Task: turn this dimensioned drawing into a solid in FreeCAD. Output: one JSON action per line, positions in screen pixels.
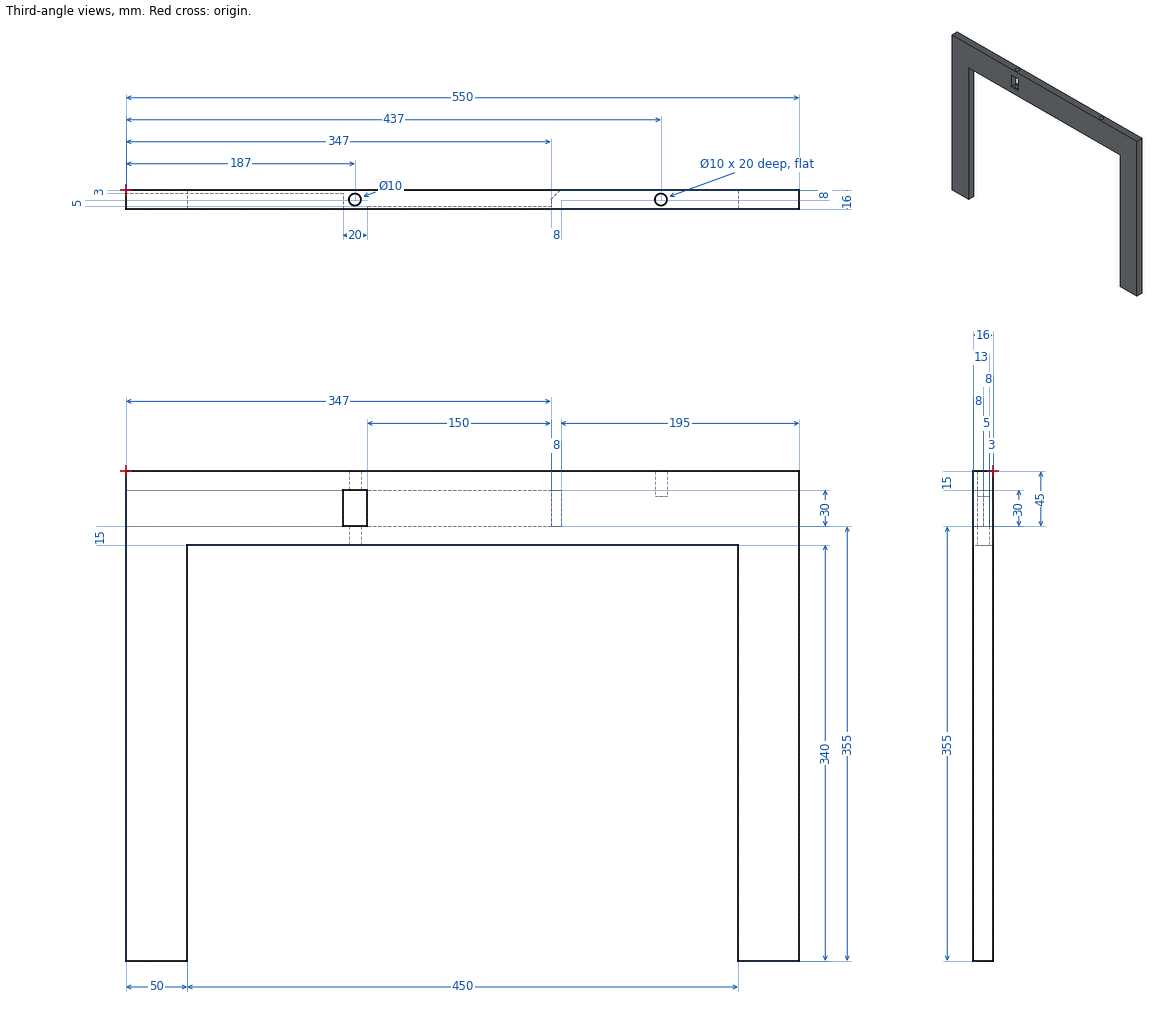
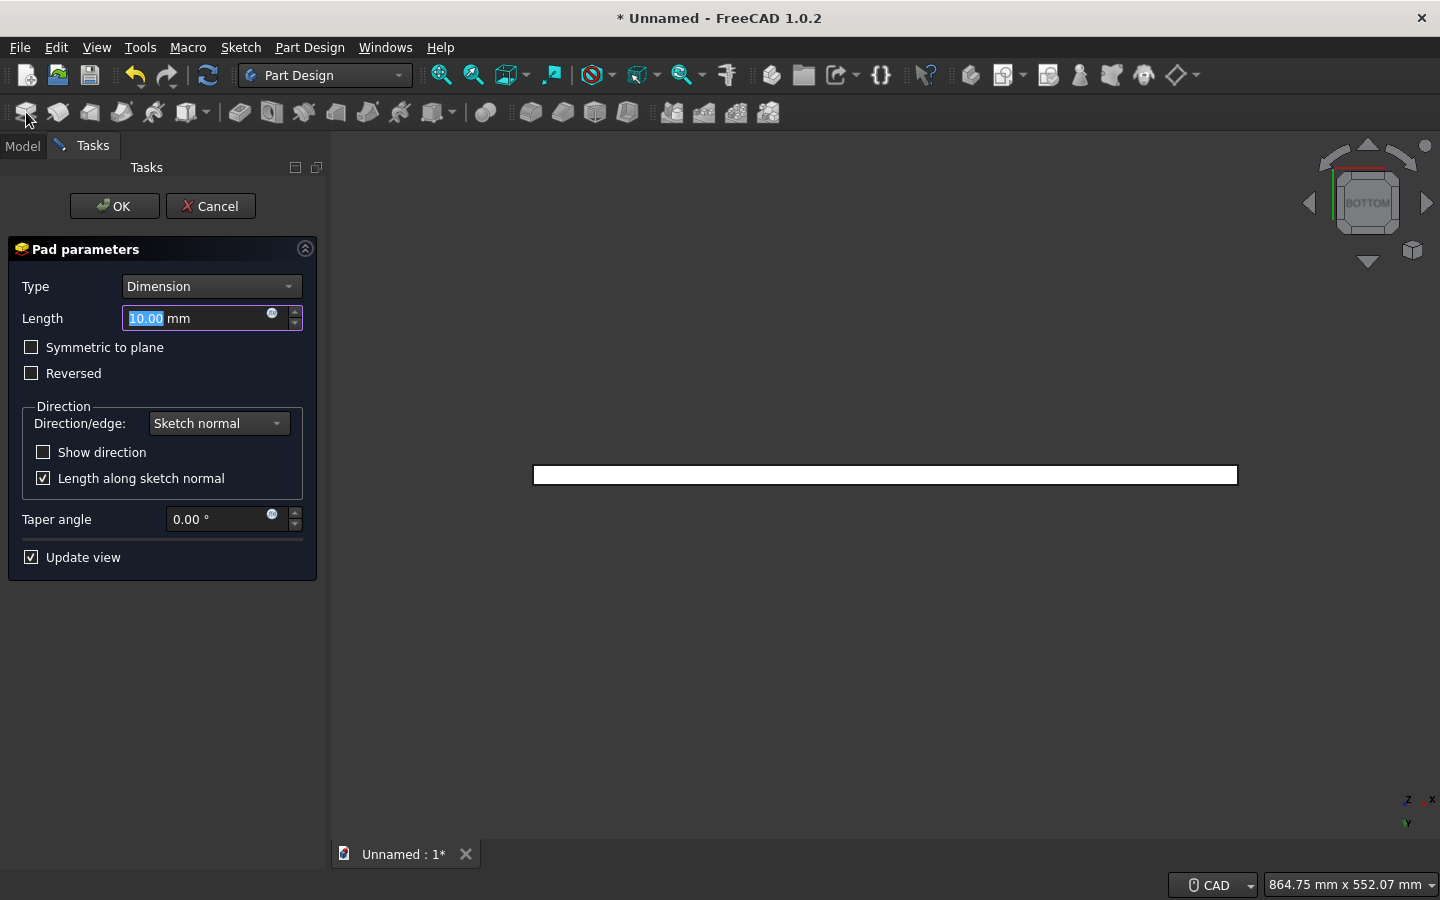
{"action": "type", "text": "355"}
{"action": "key", "text": "Tab"}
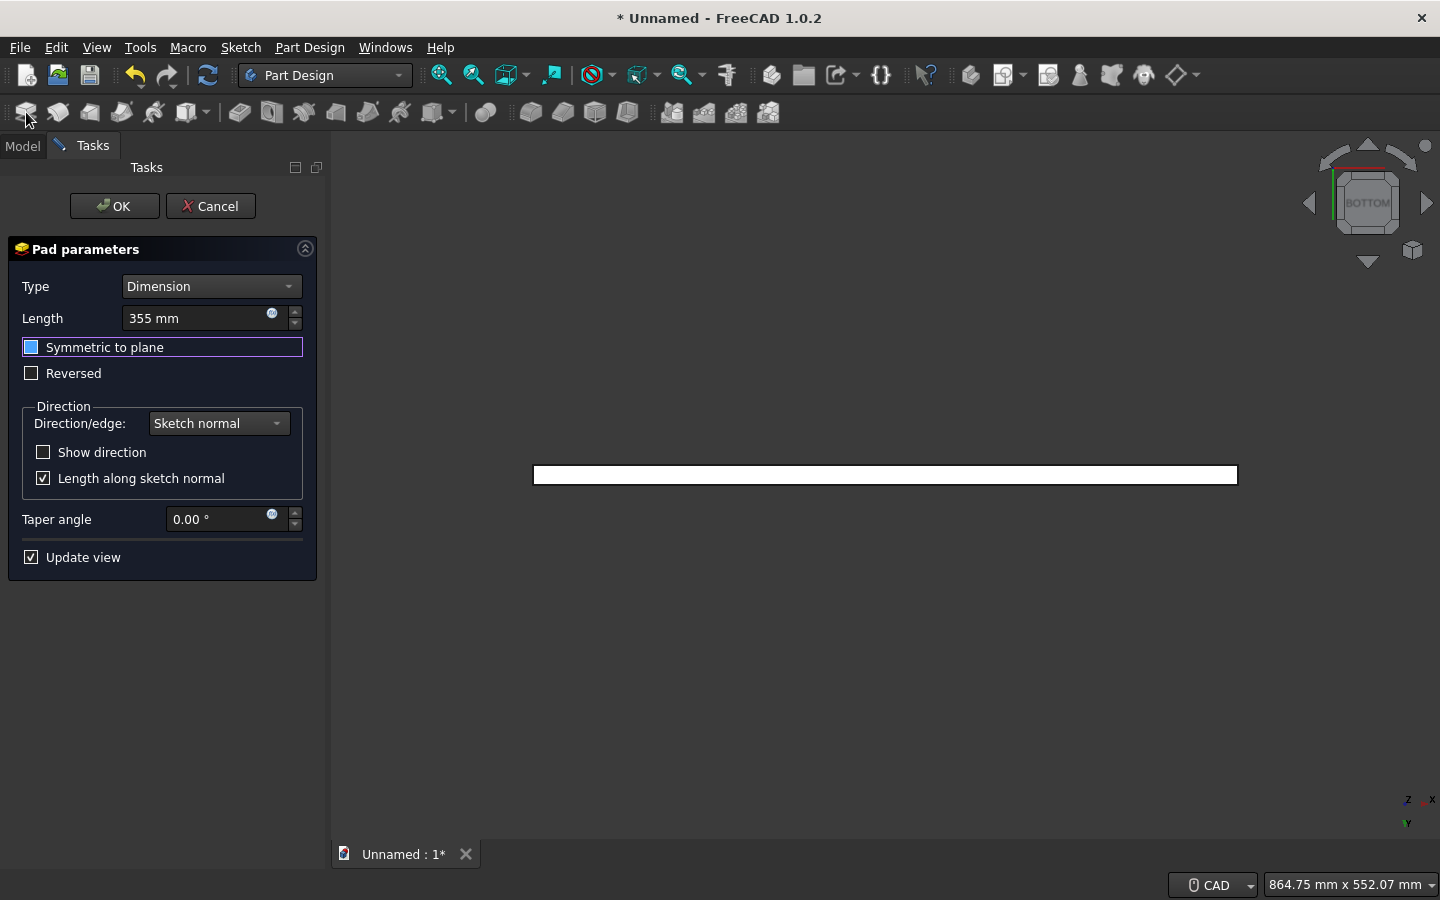
{"action": "left_click", "coordinate": [115, 206]}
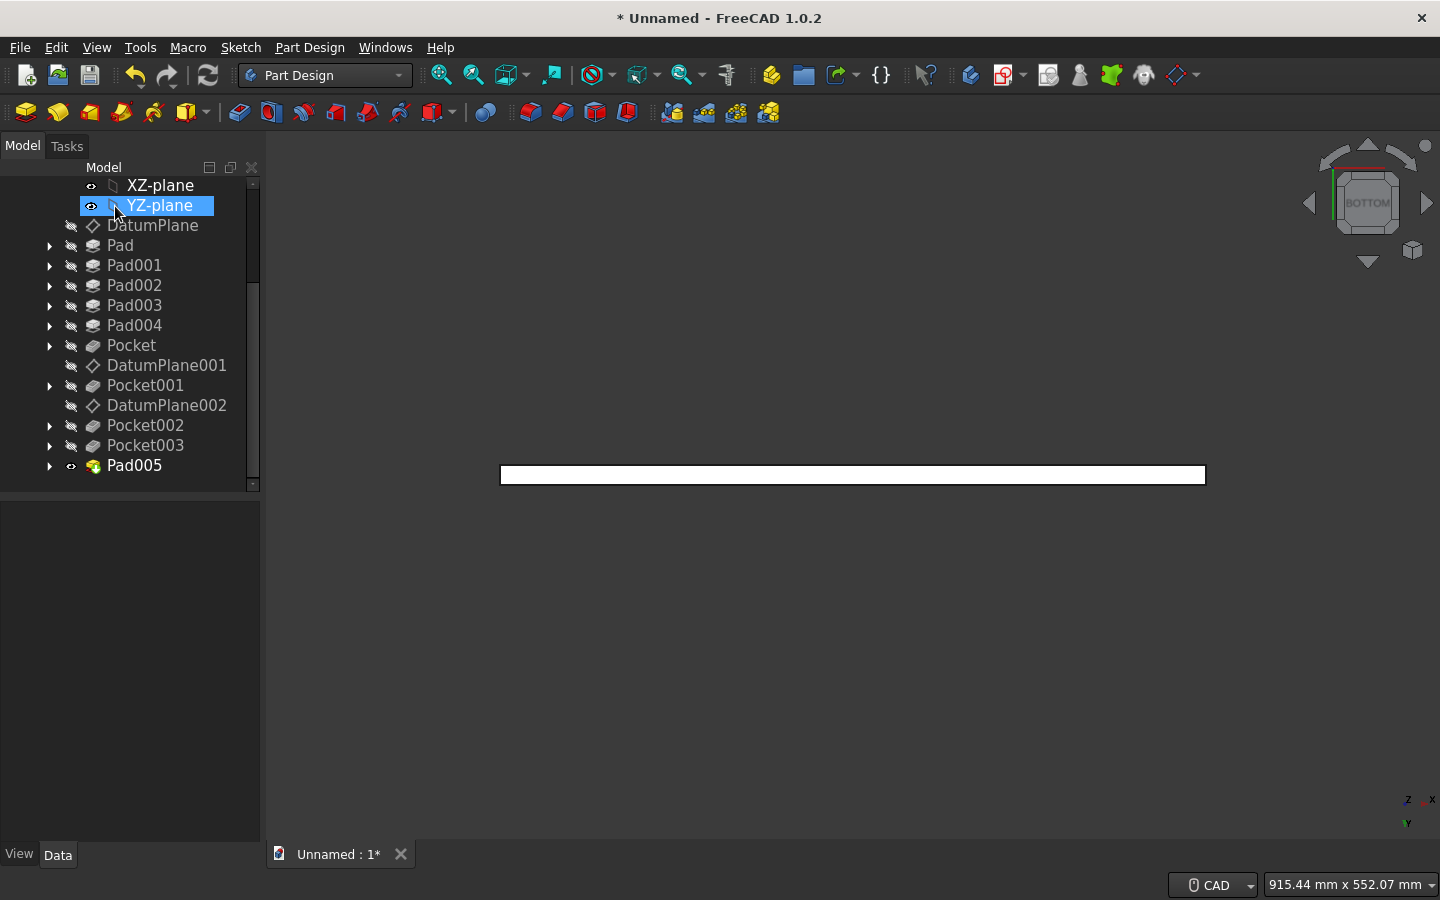
{"action": "key", "text": "4"}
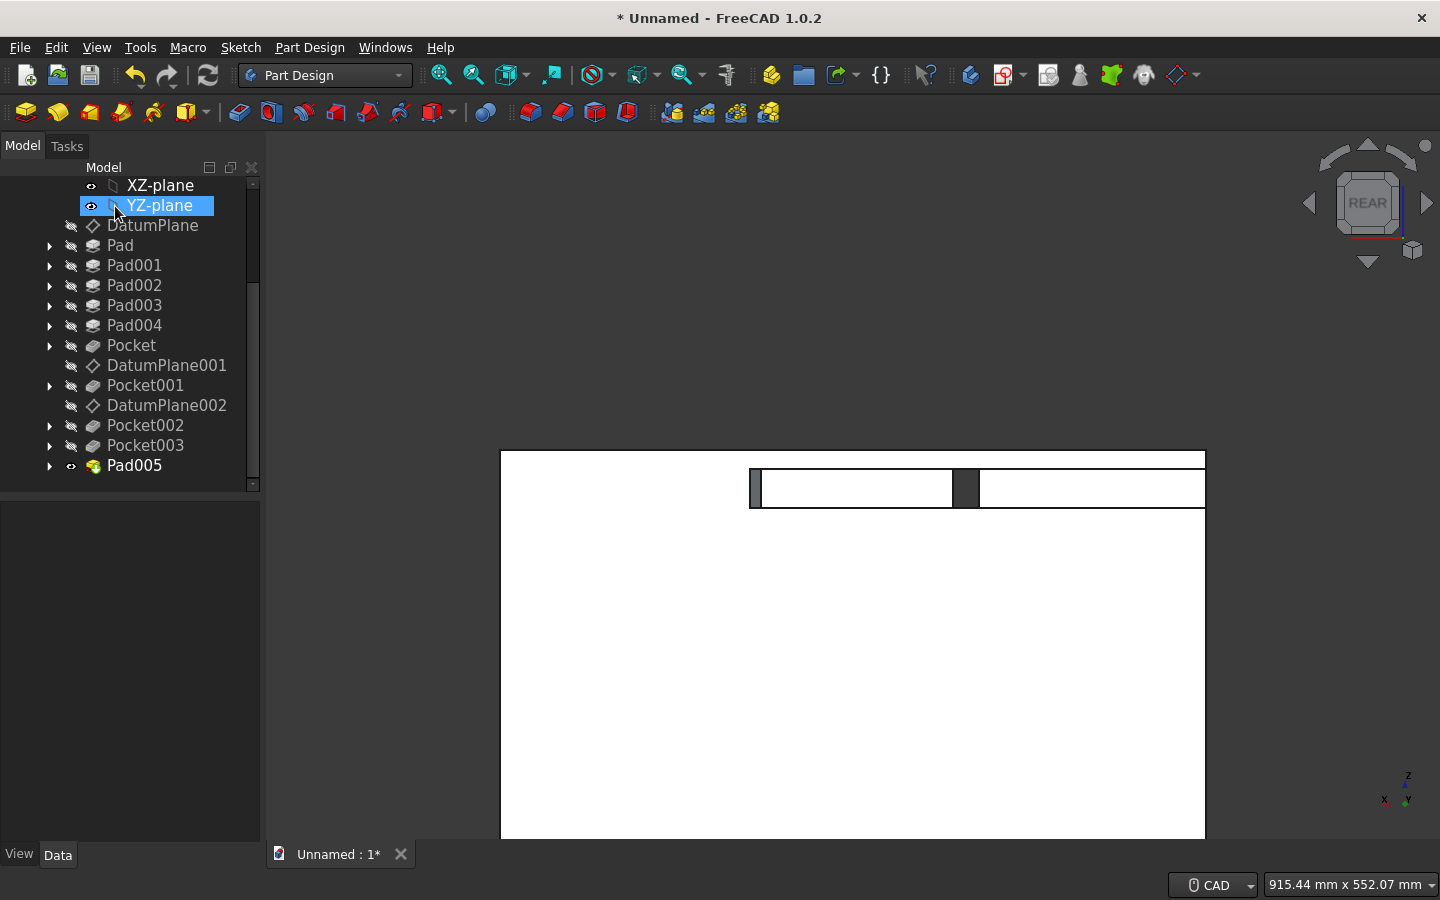
{"action": "left_click", "coordinate": [442, 76]}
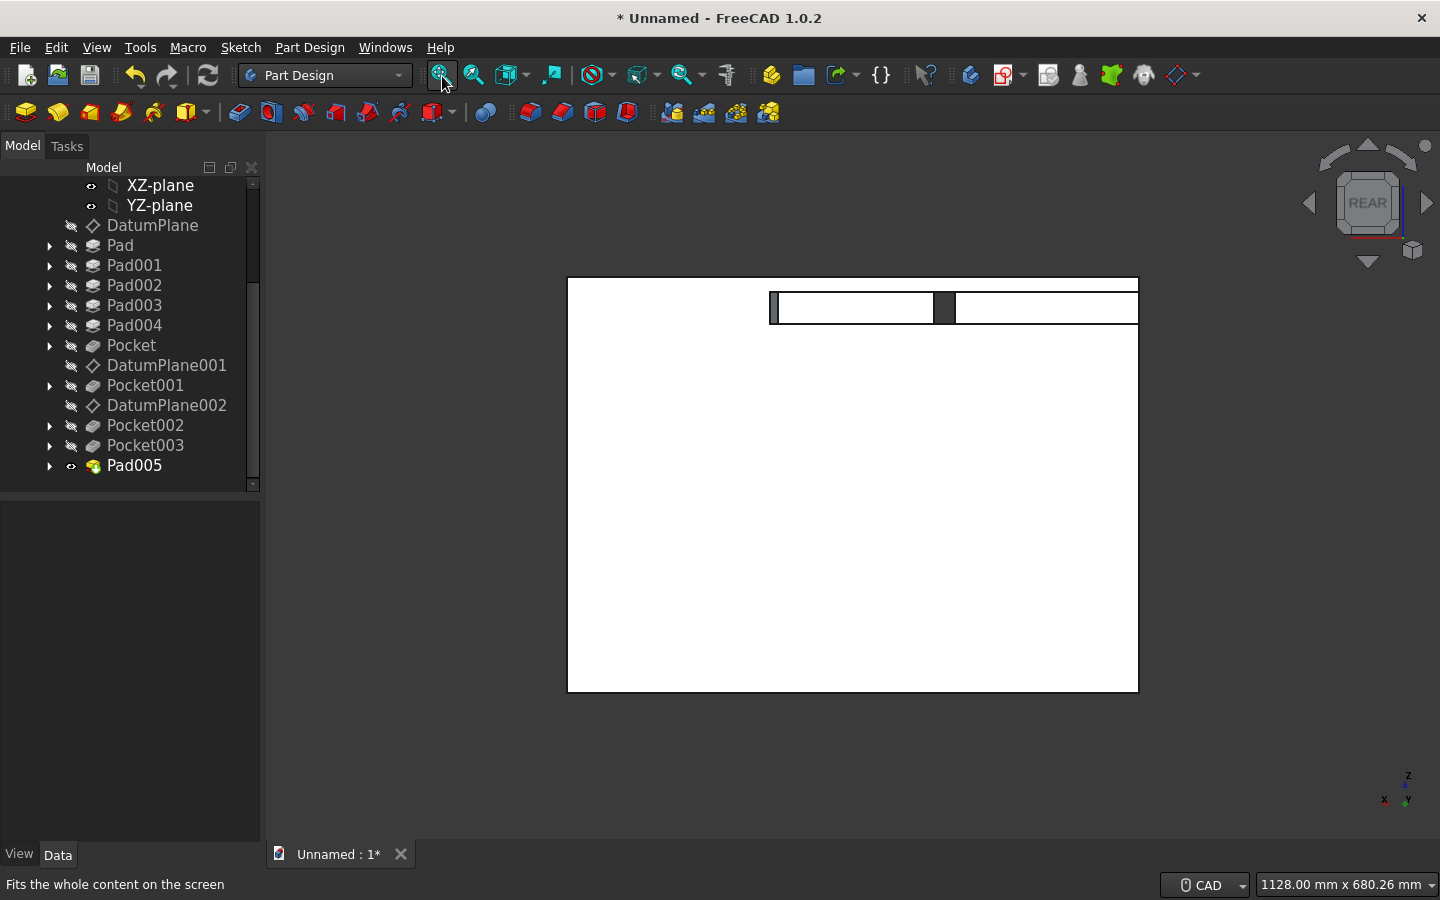
{"action": "left_click", "coordinate": [771, 484]}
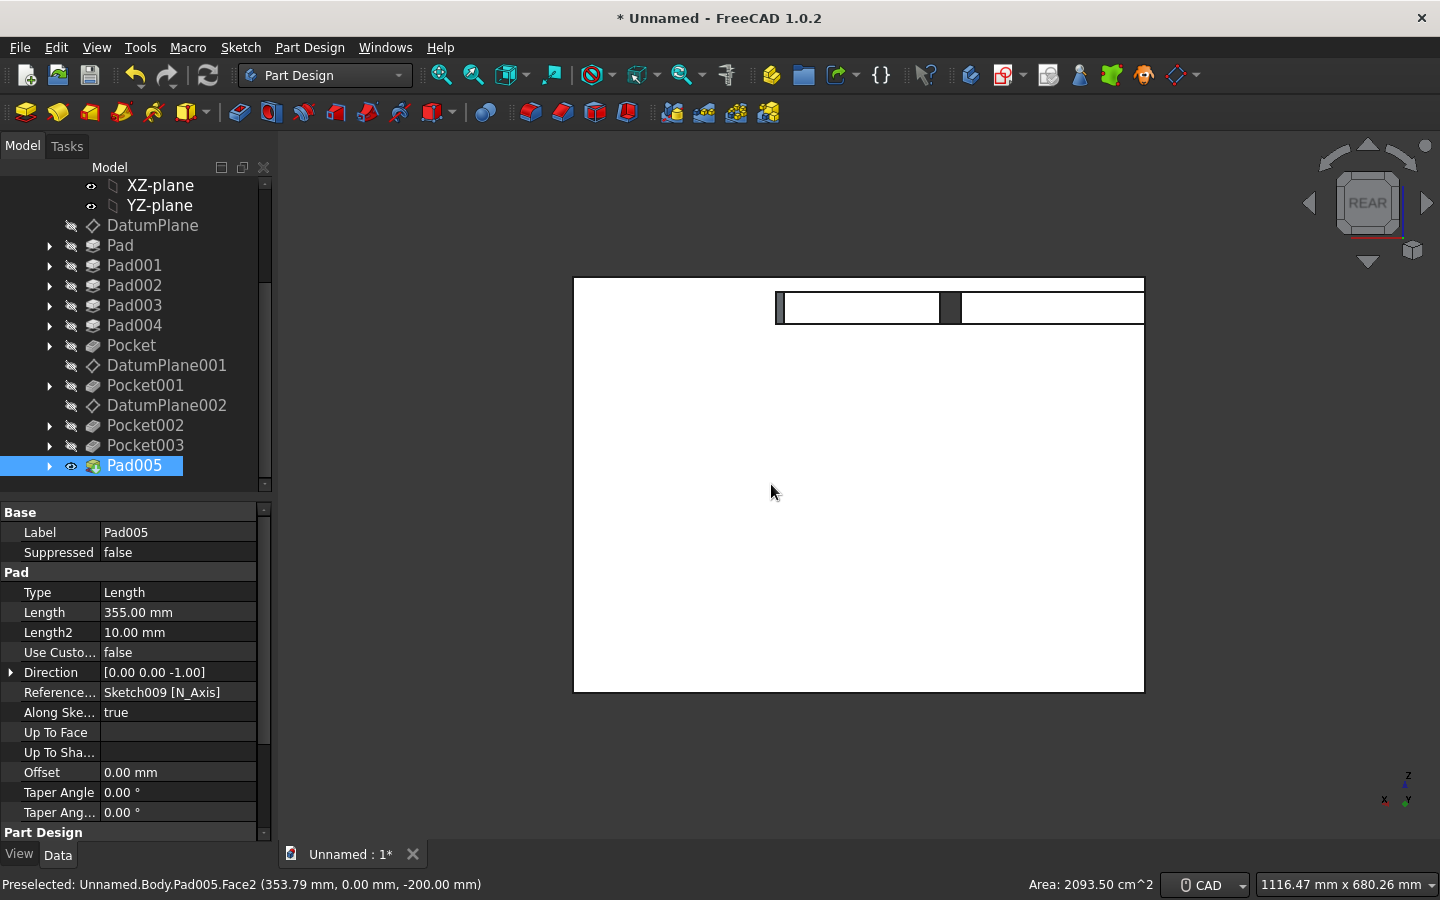
{"action": "left_click", "coordinate": [1004, 76]}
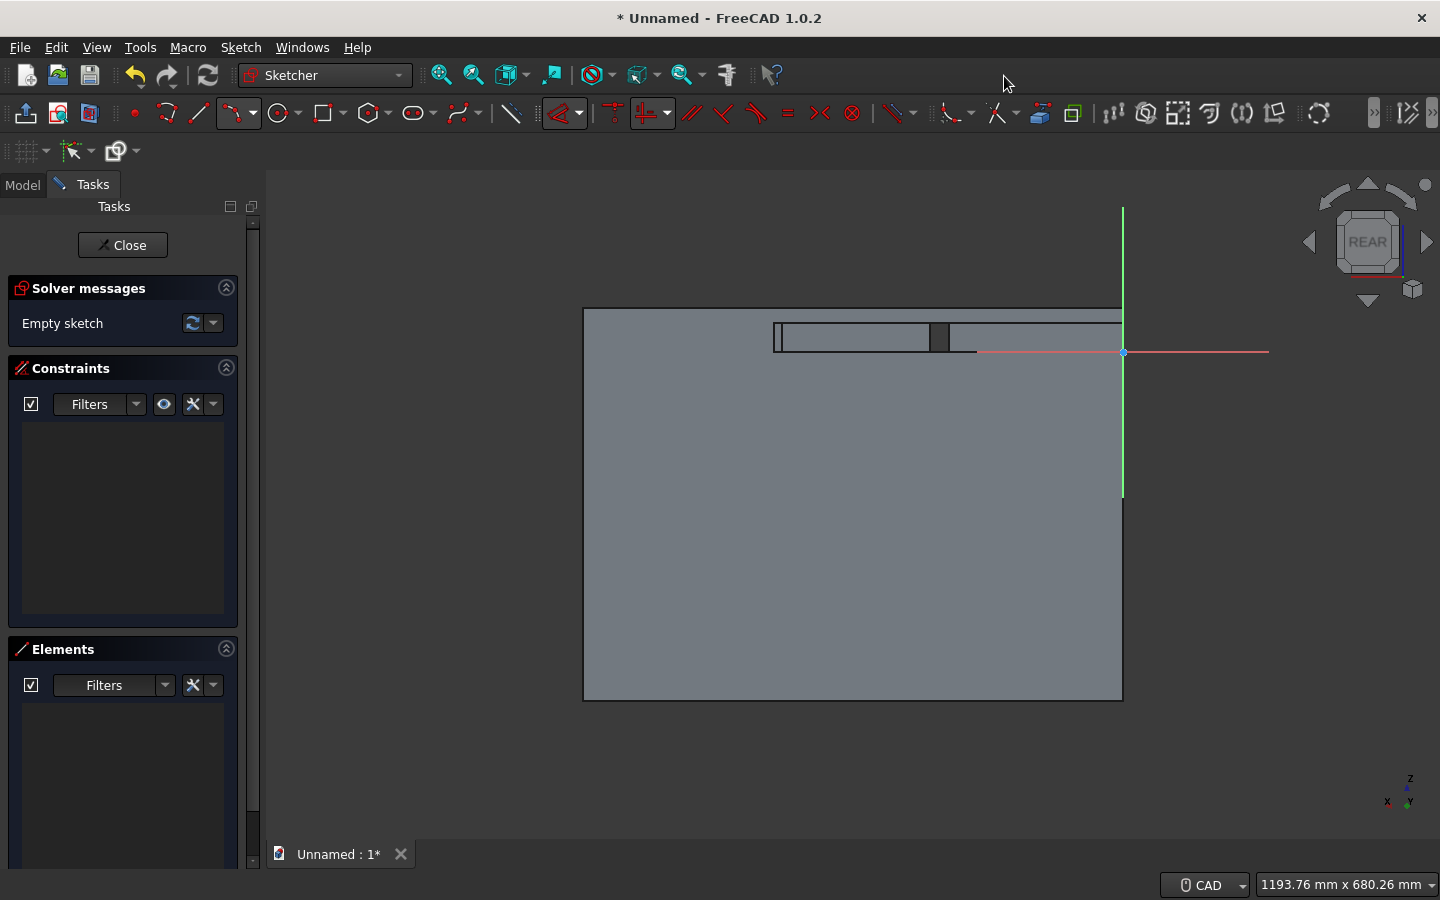
{"action": "left_click", "coordinate": [324, 114]}